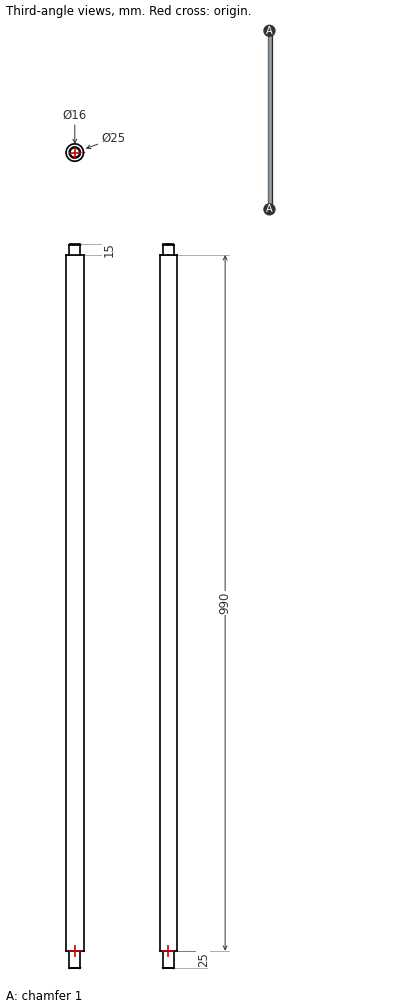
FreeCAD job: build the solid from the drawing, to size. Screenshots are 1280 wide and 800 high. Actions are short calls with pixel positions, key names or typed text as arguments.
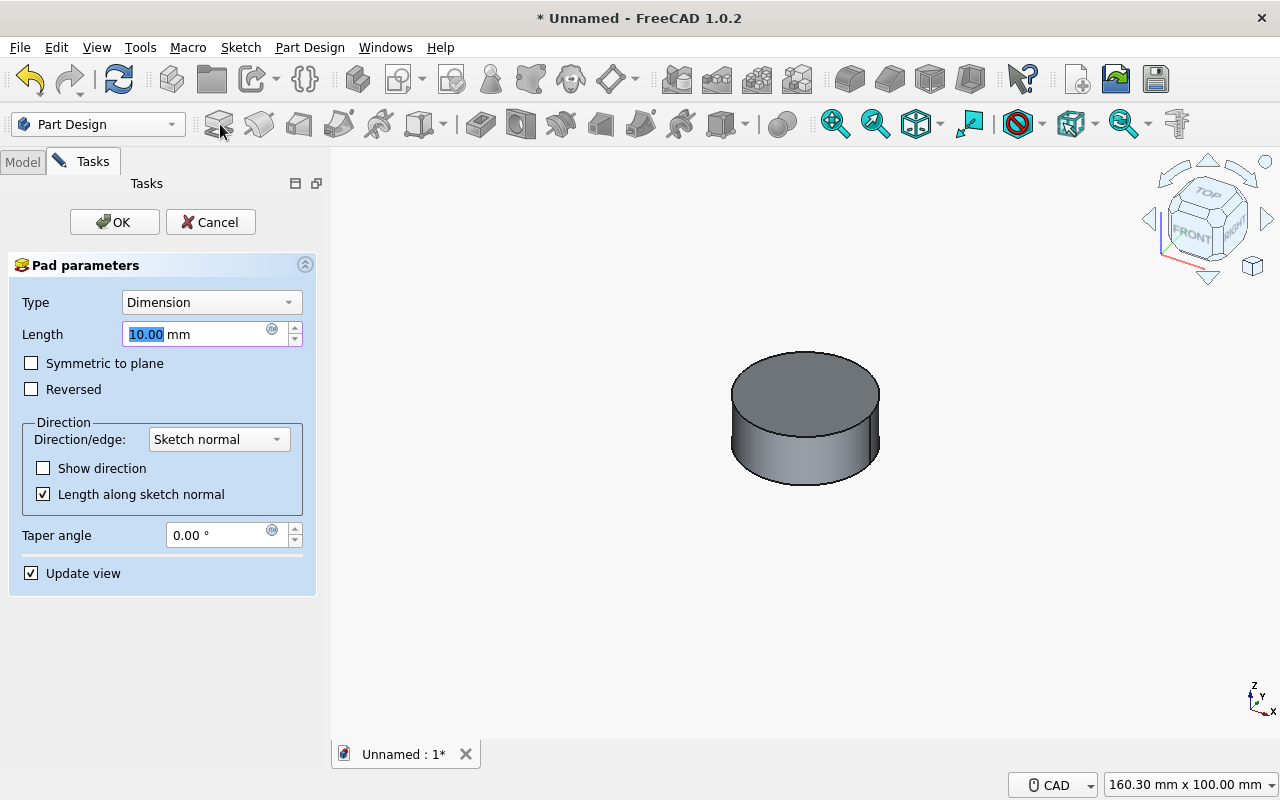
text(990)
key(Tab)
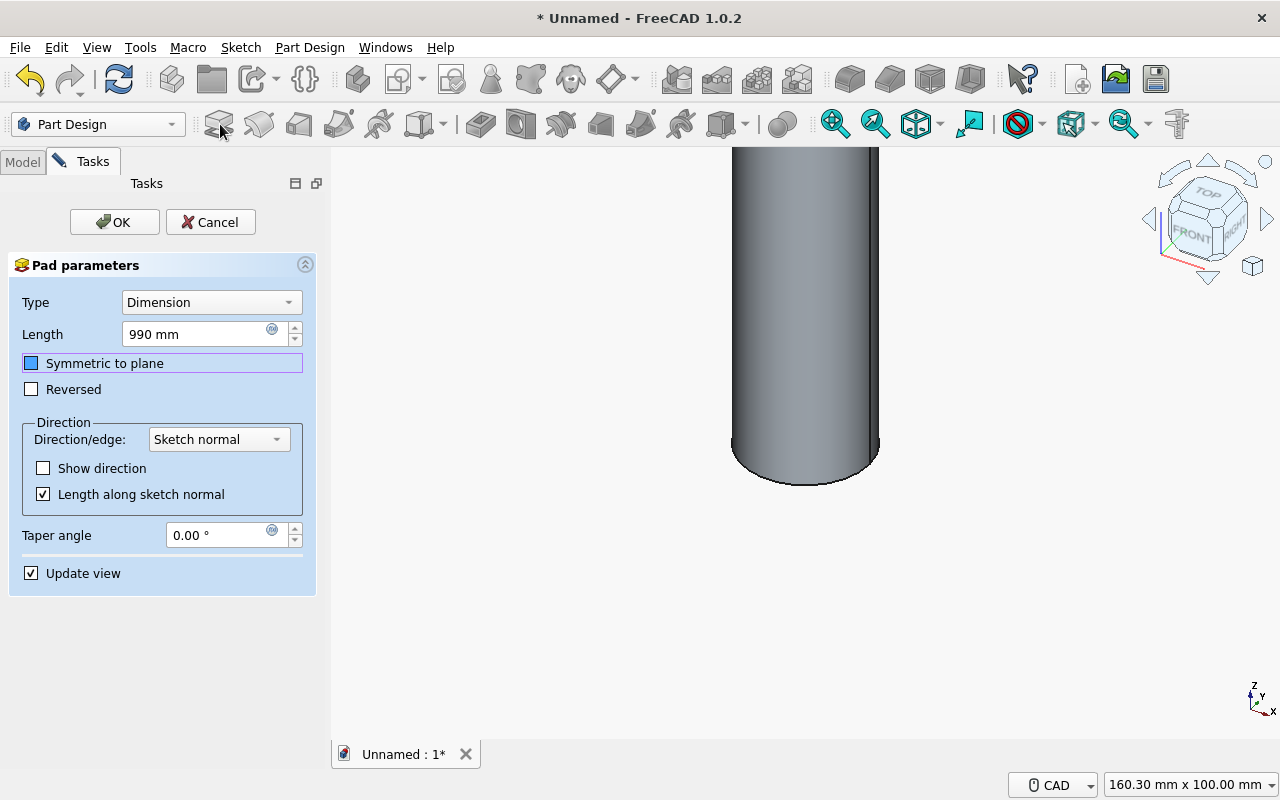
click(115, 222)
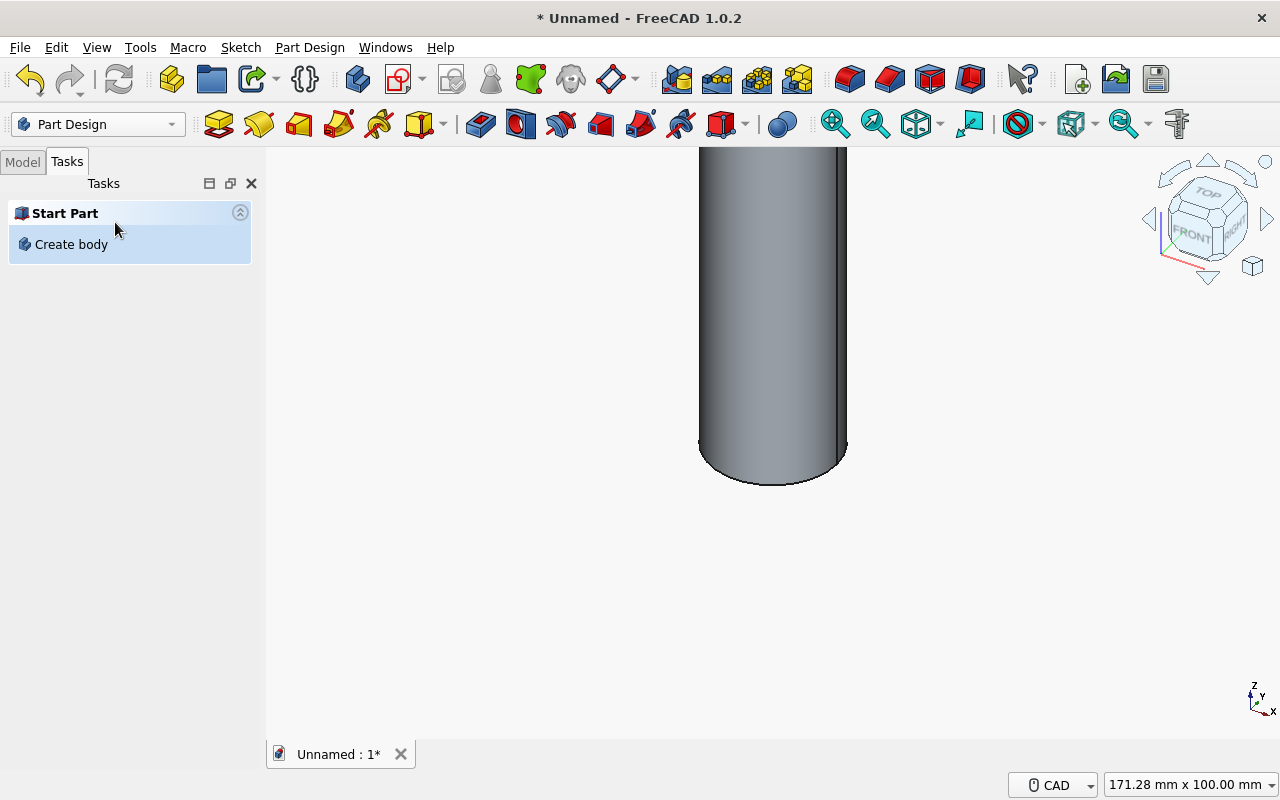
click(836, 124)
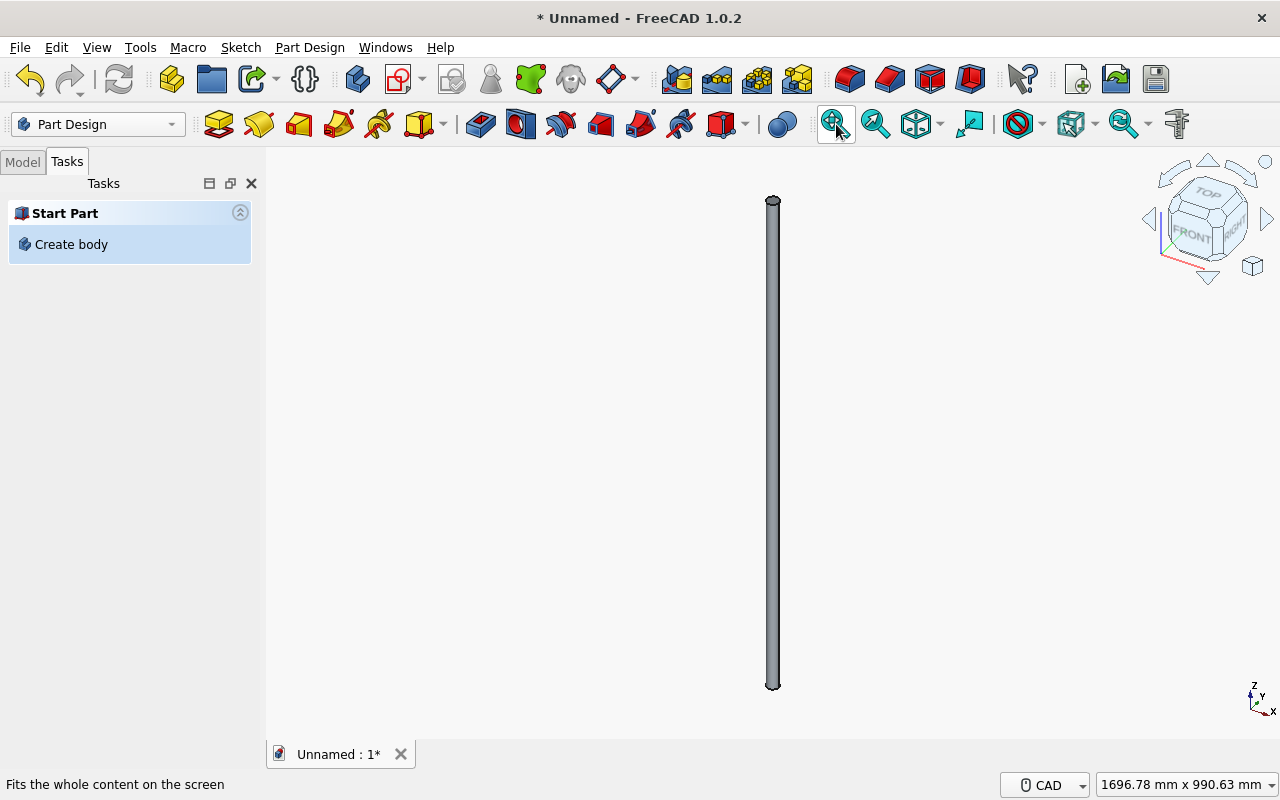
key(0)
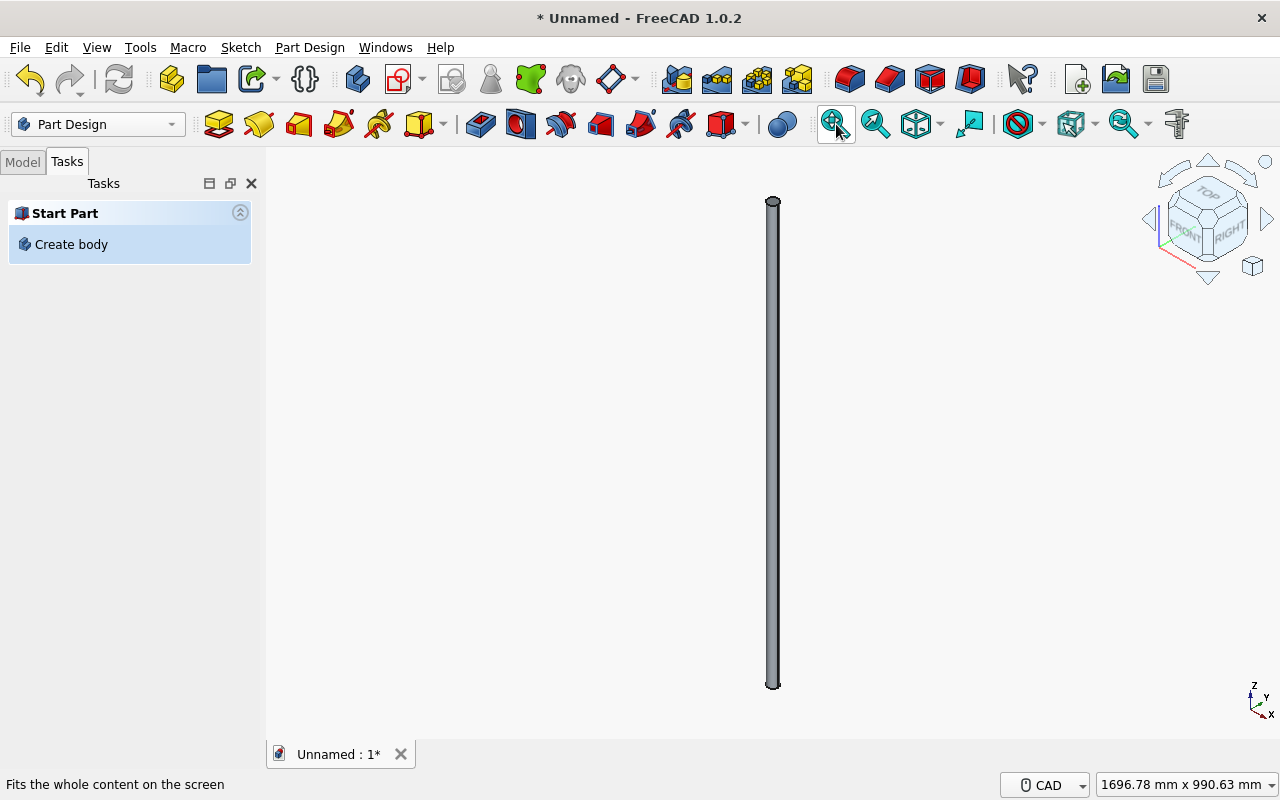
key(2)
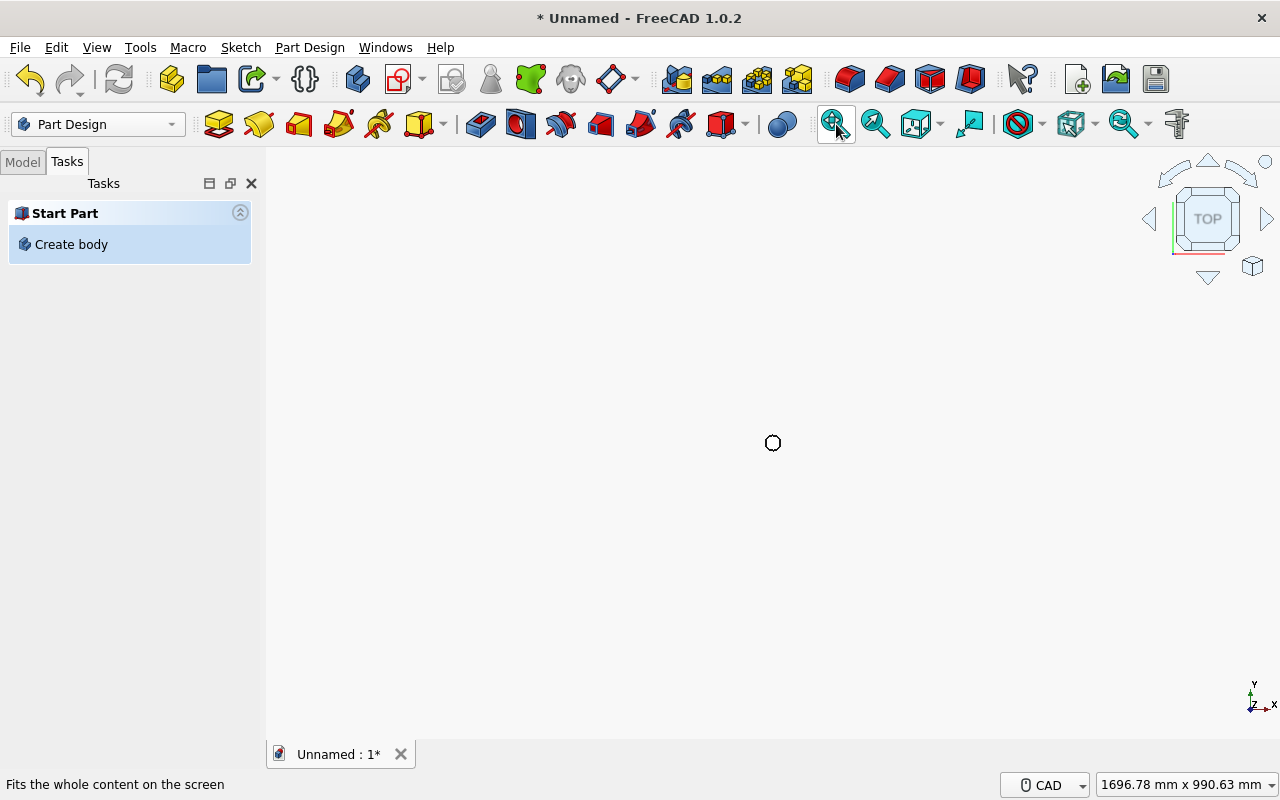
click(836, 124)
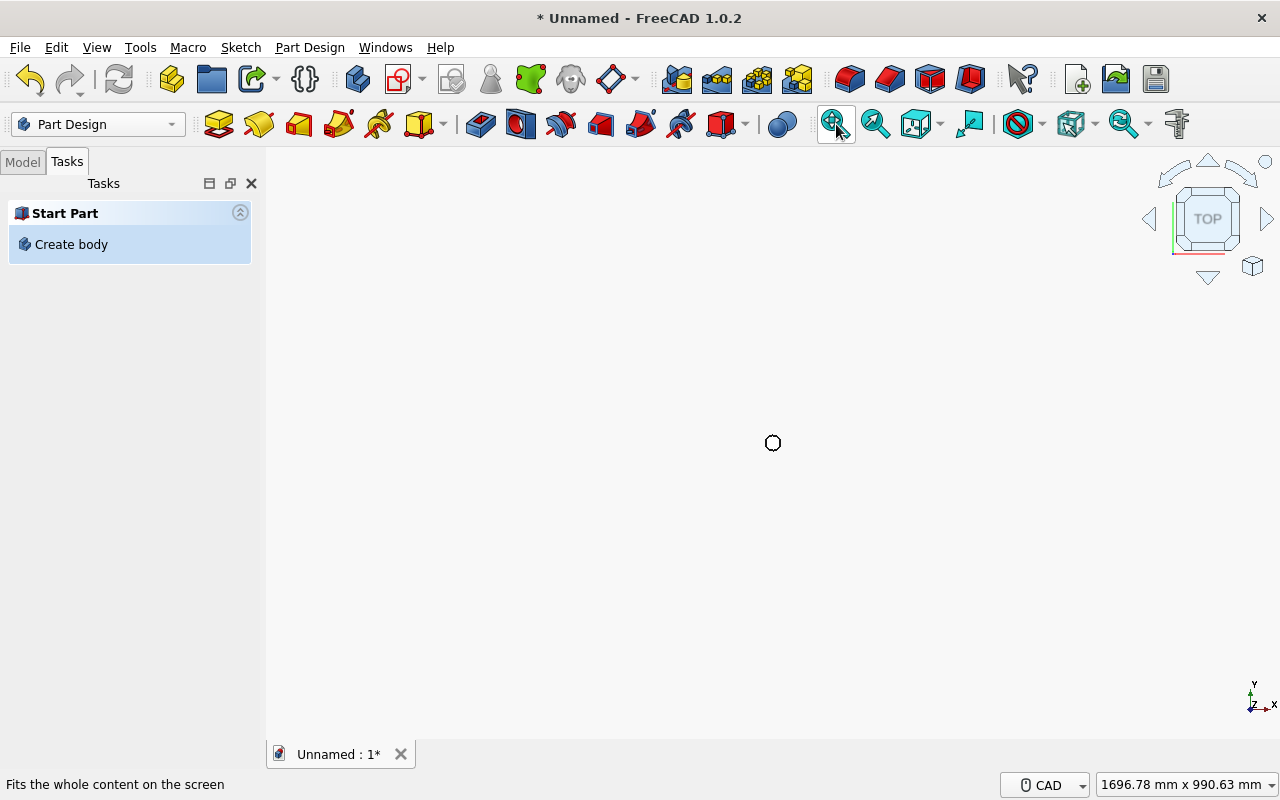
key(1)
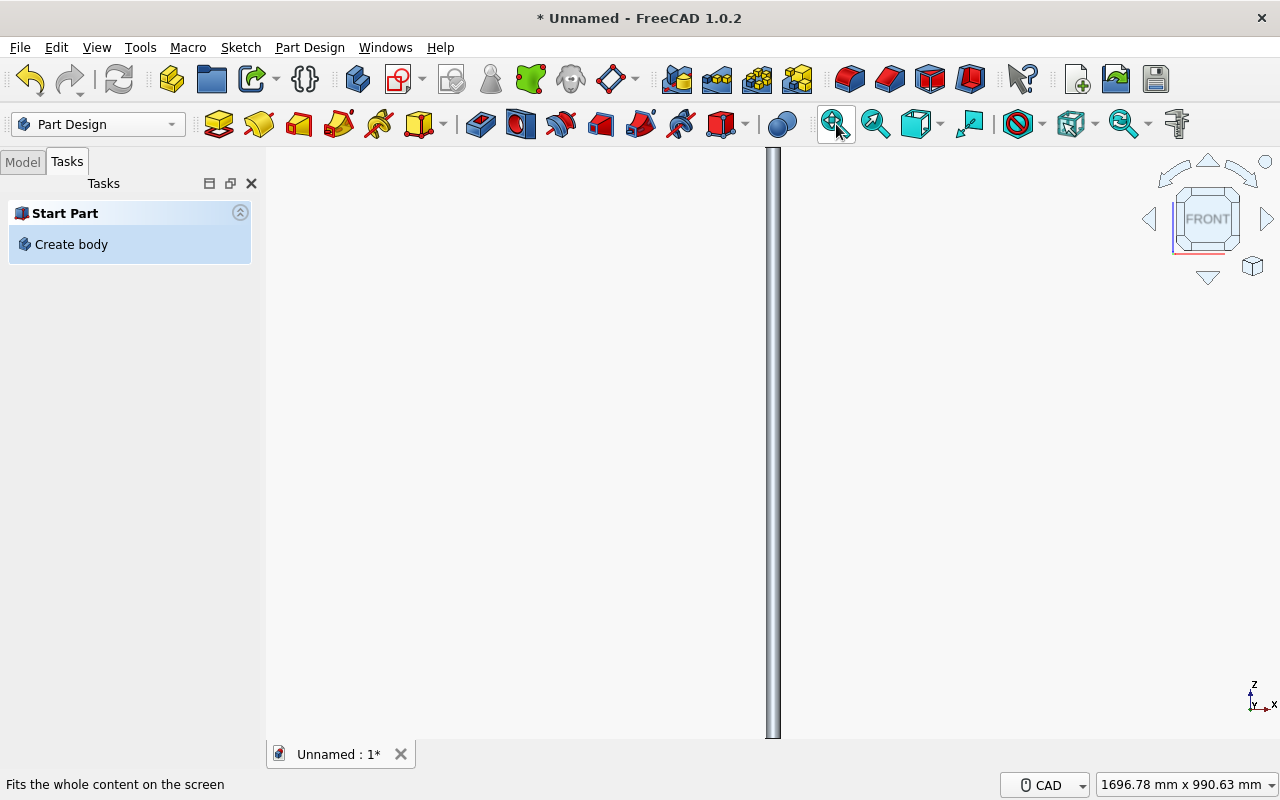
click(836, 124)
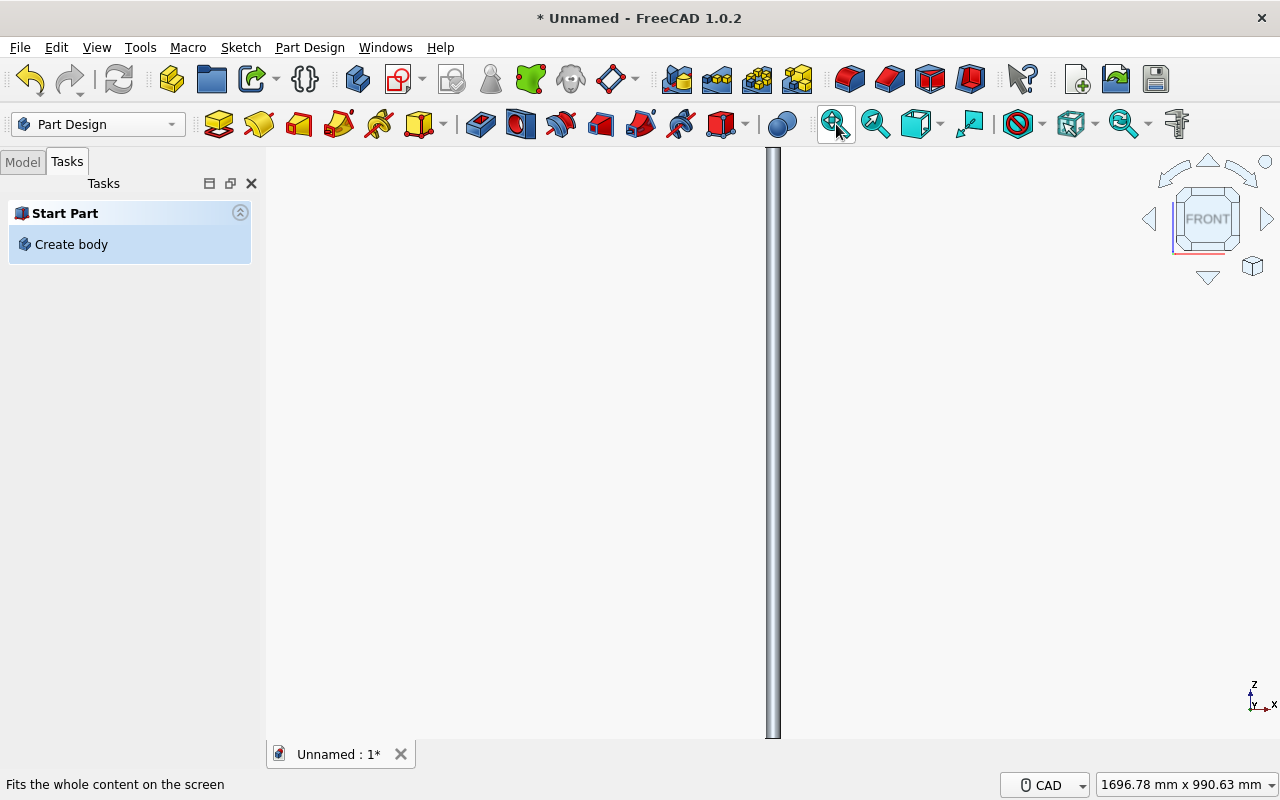
click(23, 161)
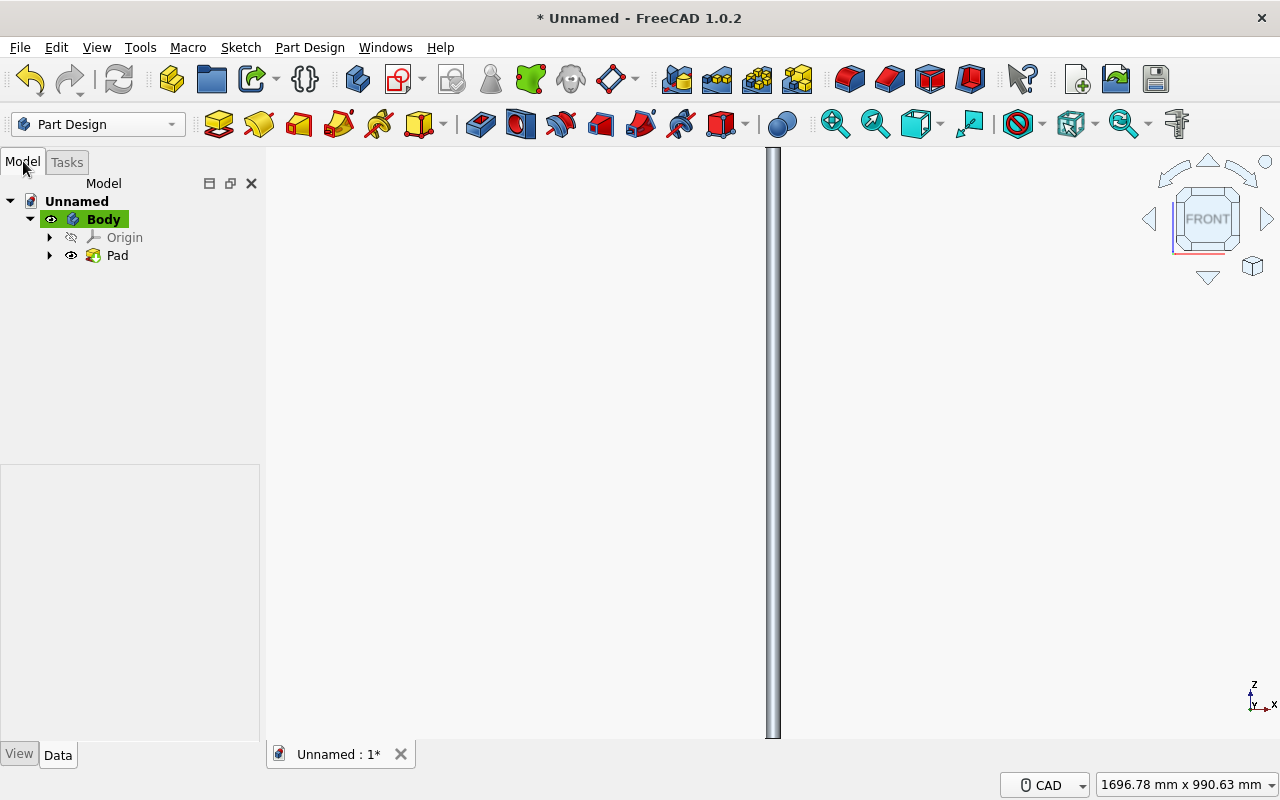
click(50, 237)